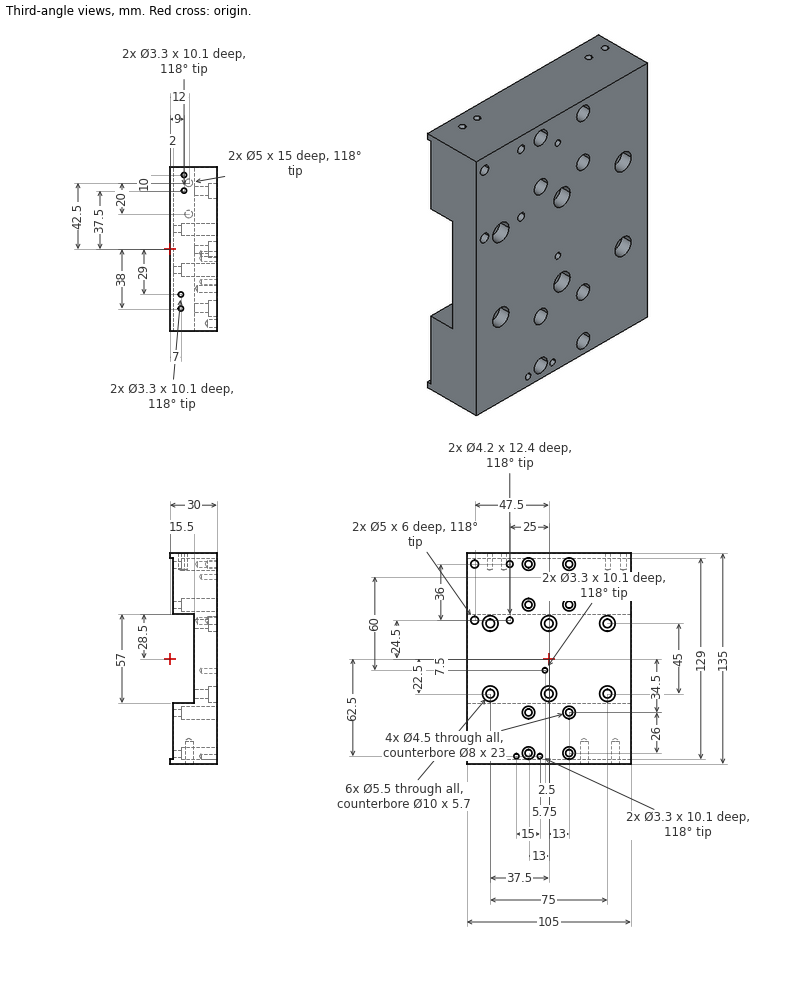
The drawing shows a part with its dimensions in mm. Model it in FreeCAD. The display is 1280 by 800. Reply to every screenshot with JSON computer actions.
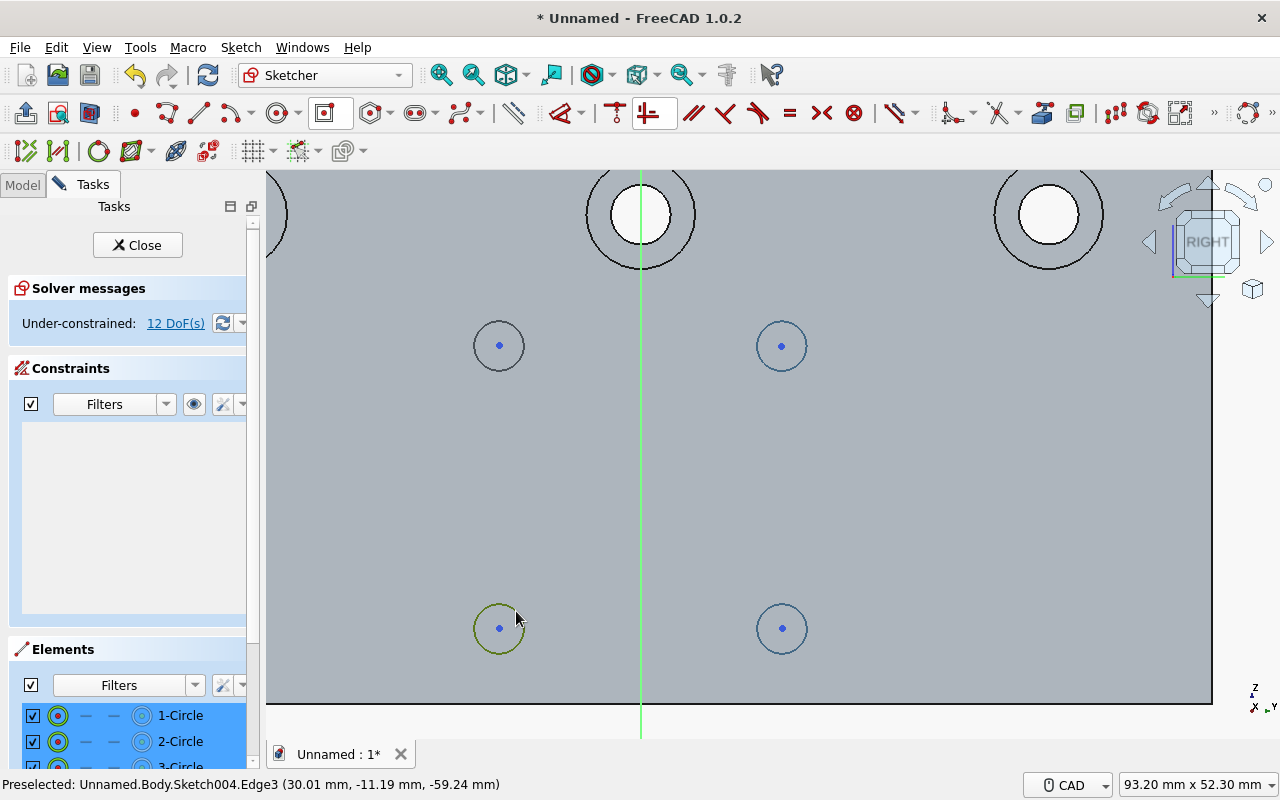
{"action": "left_click", "coordinate": [516, 328]}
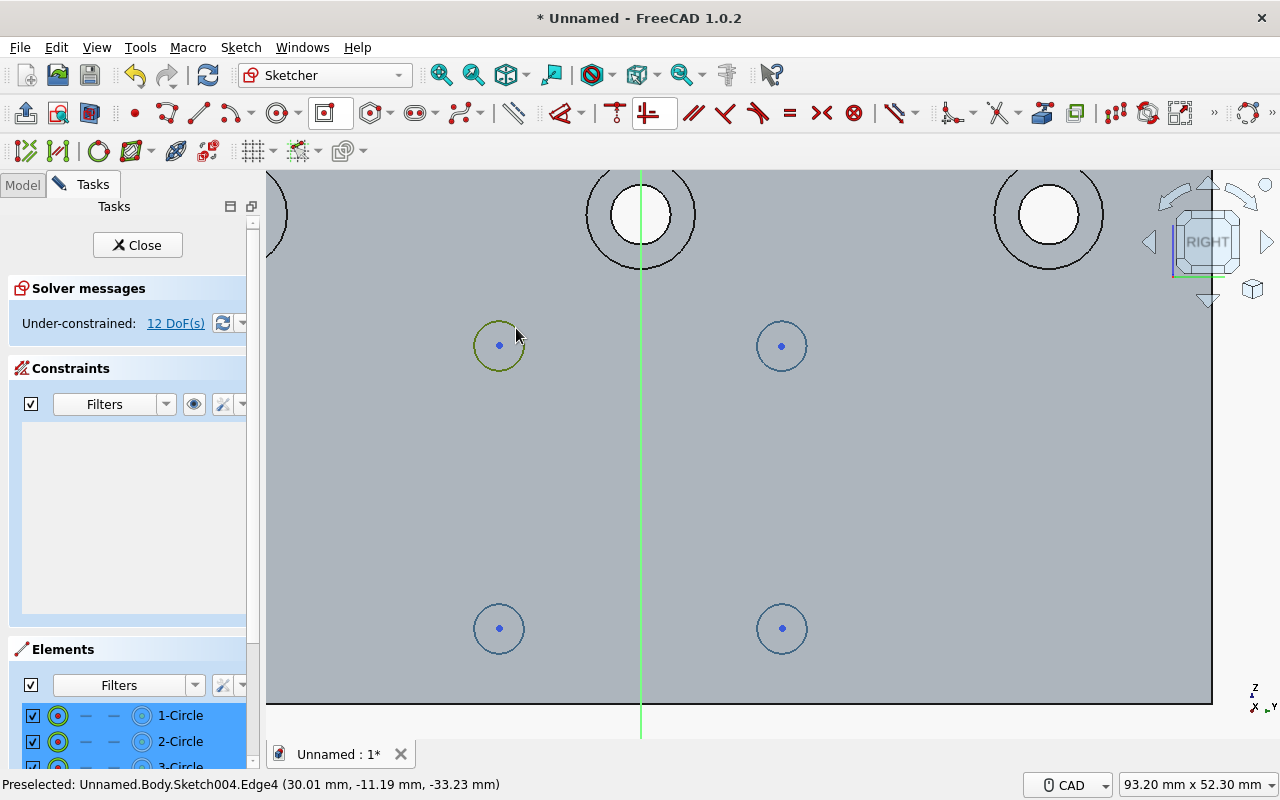
{"action": "left_click", "coordinate": [790, 114]}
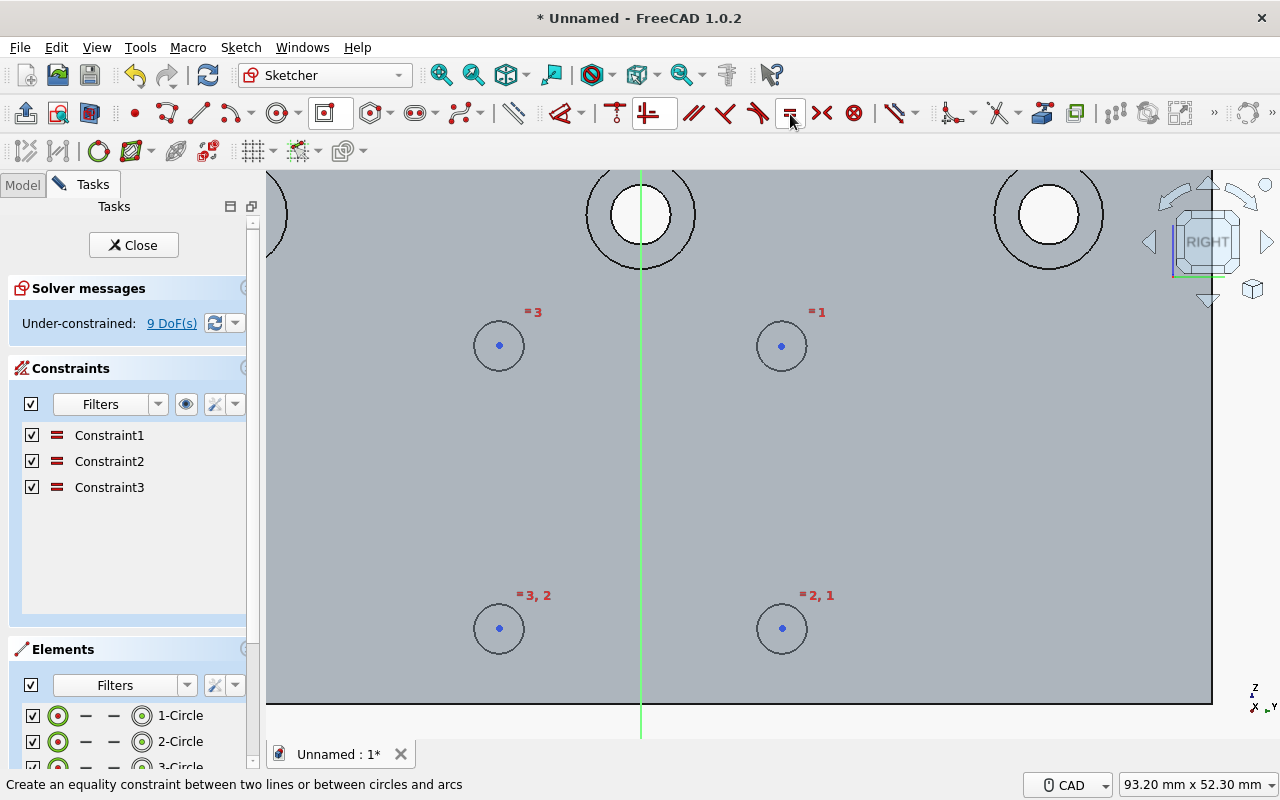
{"action": "left_click", "coordinate": [782, 346]}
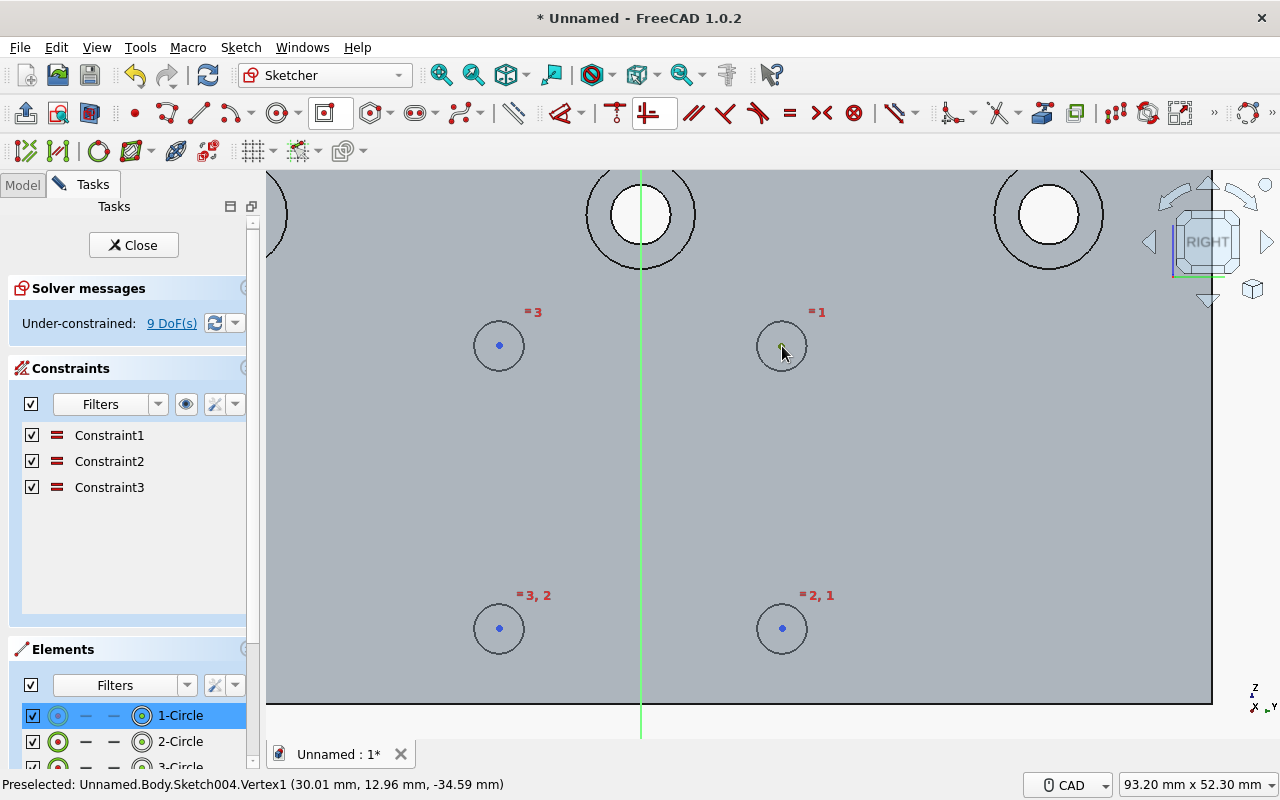
{"action": "left_click", "coordinate": [782, 629]}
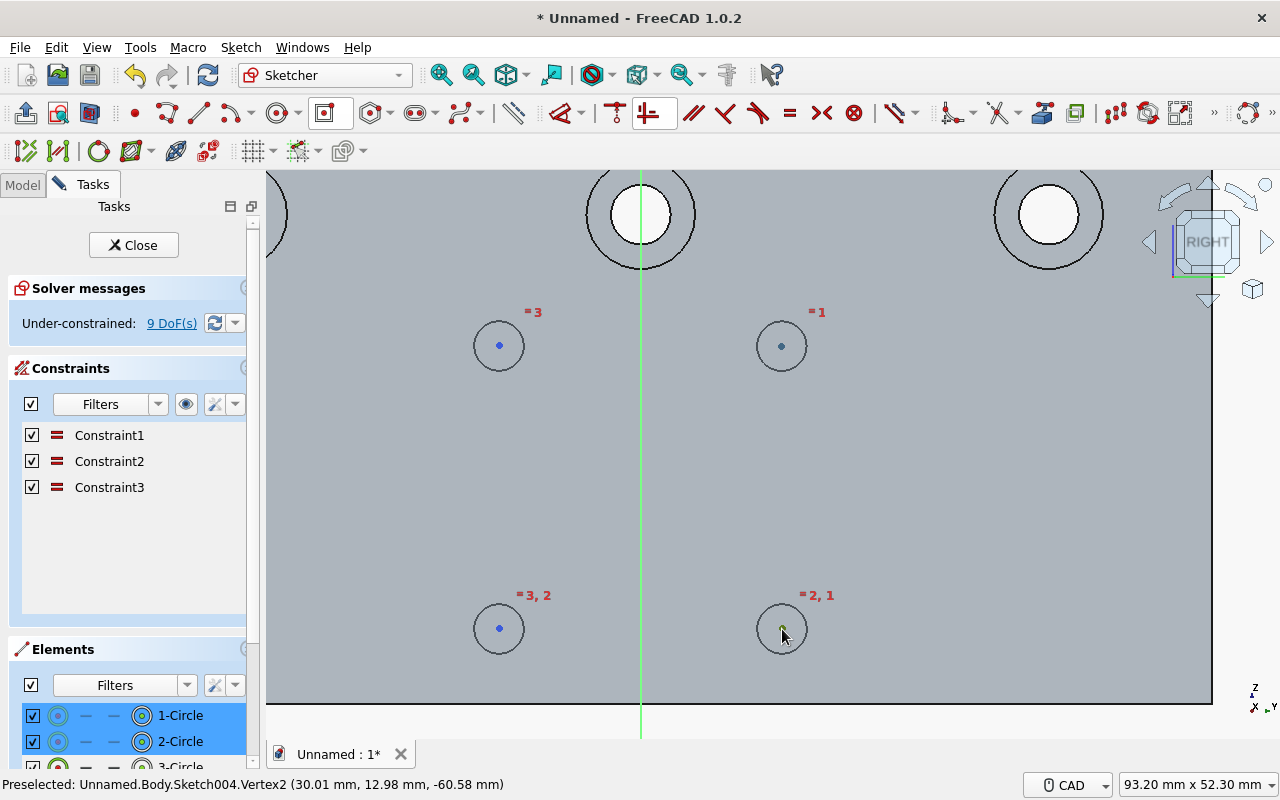
{"action": "left_click", "coordinate": [672, 114]}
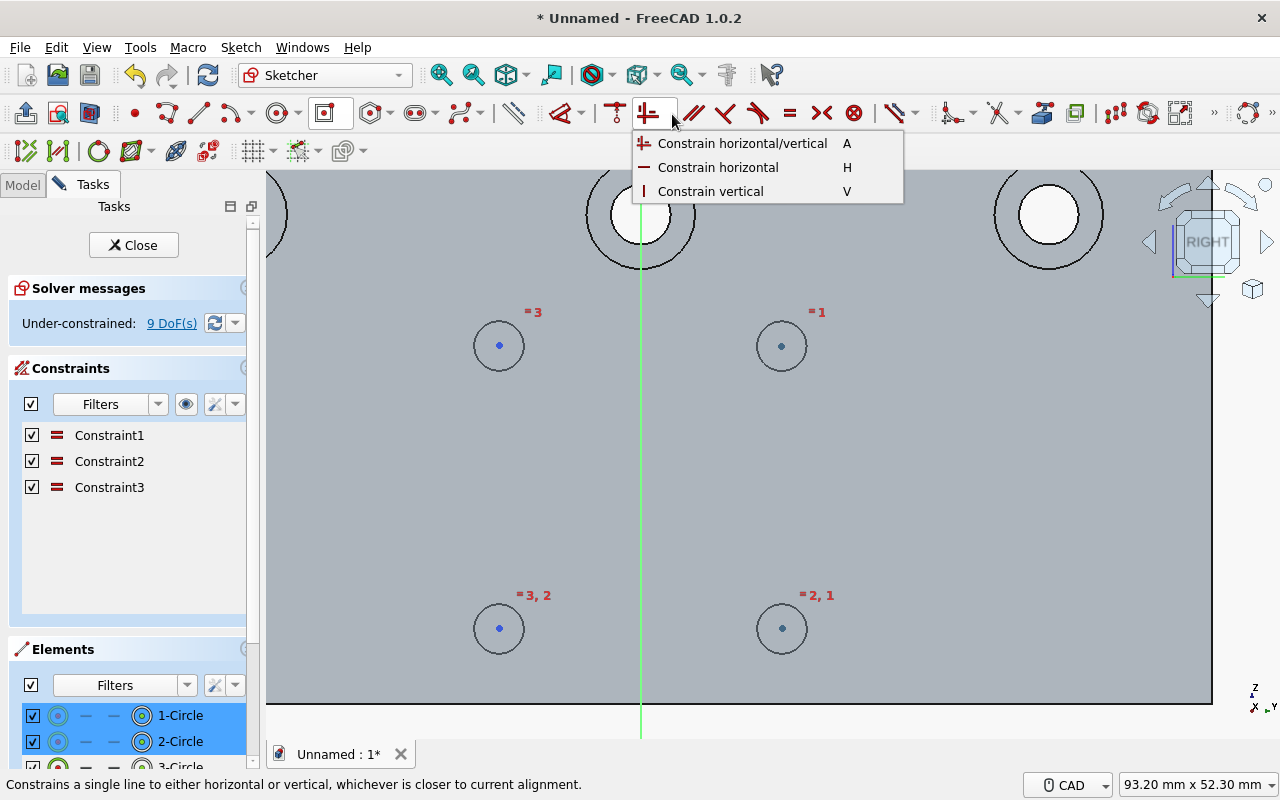
{"action": "left_click", "coordinate": [768, 191]}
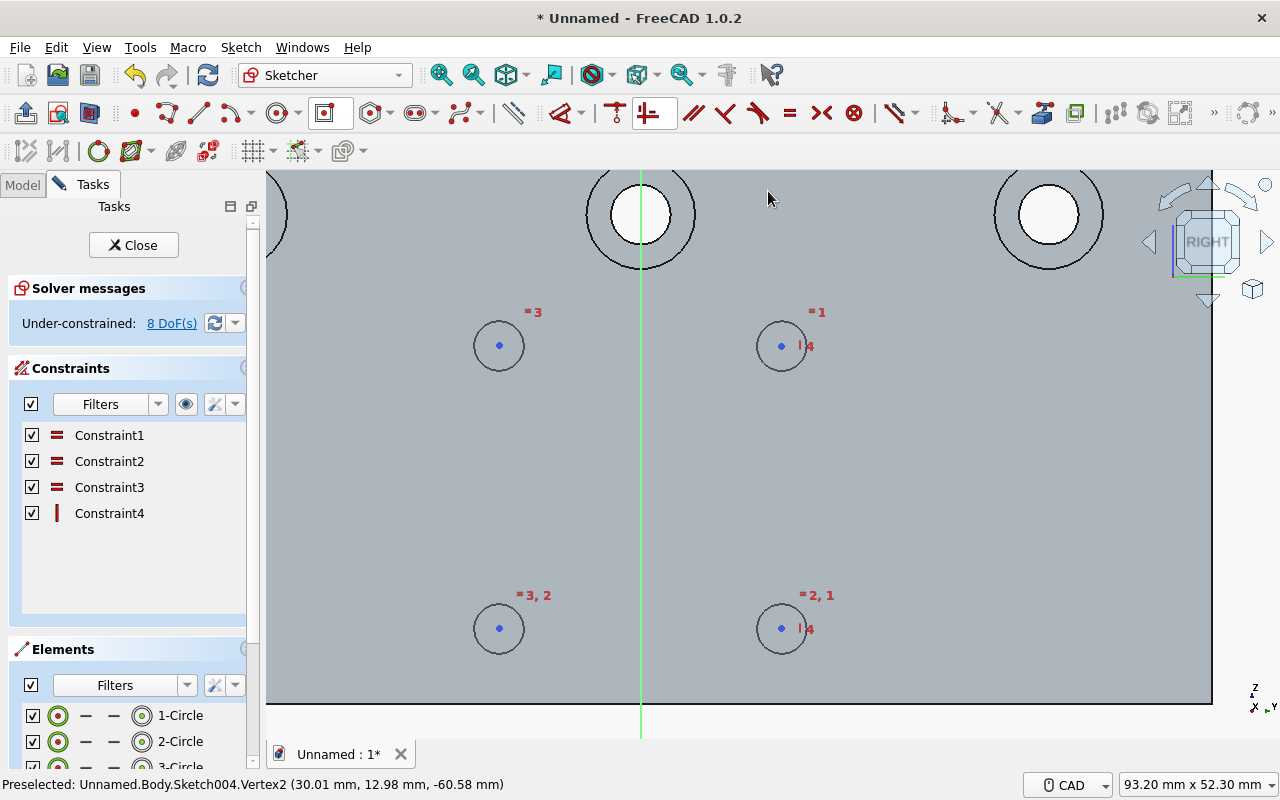
{"action": "left_click", "coordinate": [782, 629]}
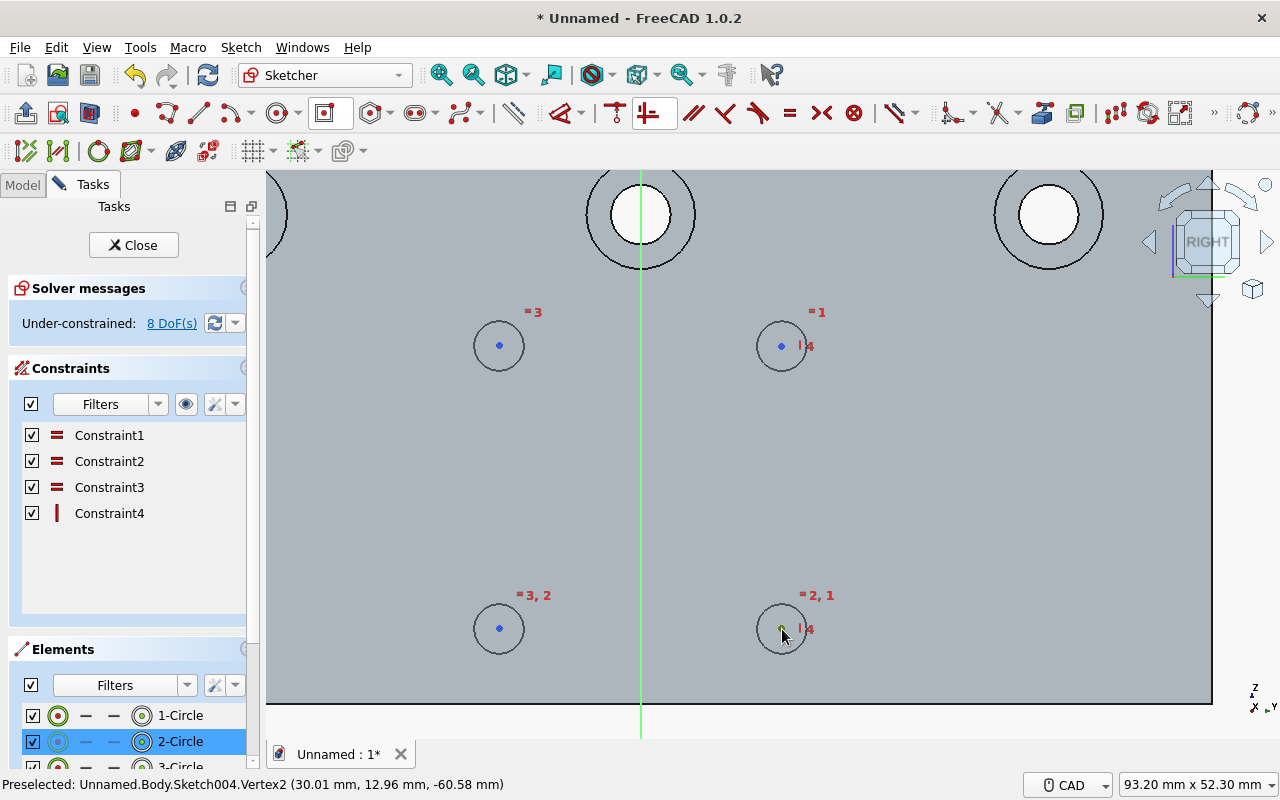
{"action": "left_click", "coordinate": [499, 629]}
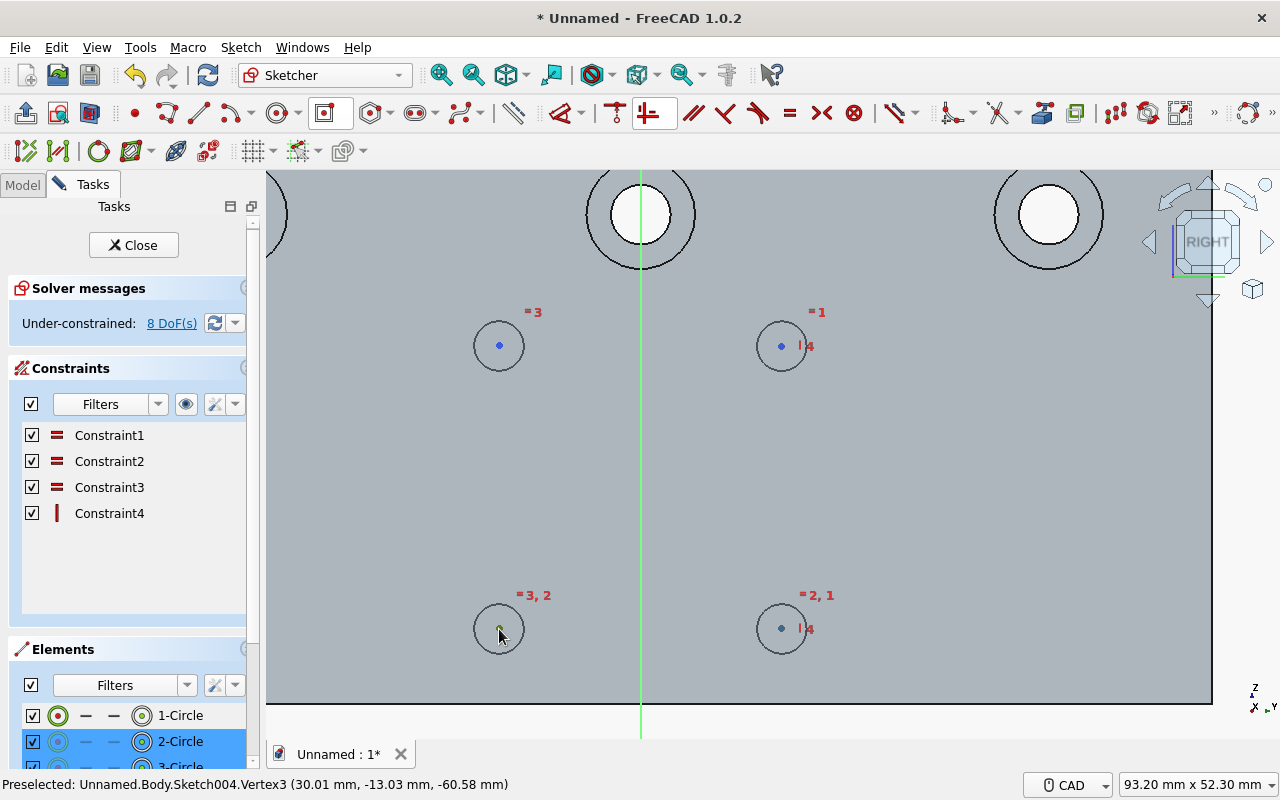
{"action": "key", "text": "h"}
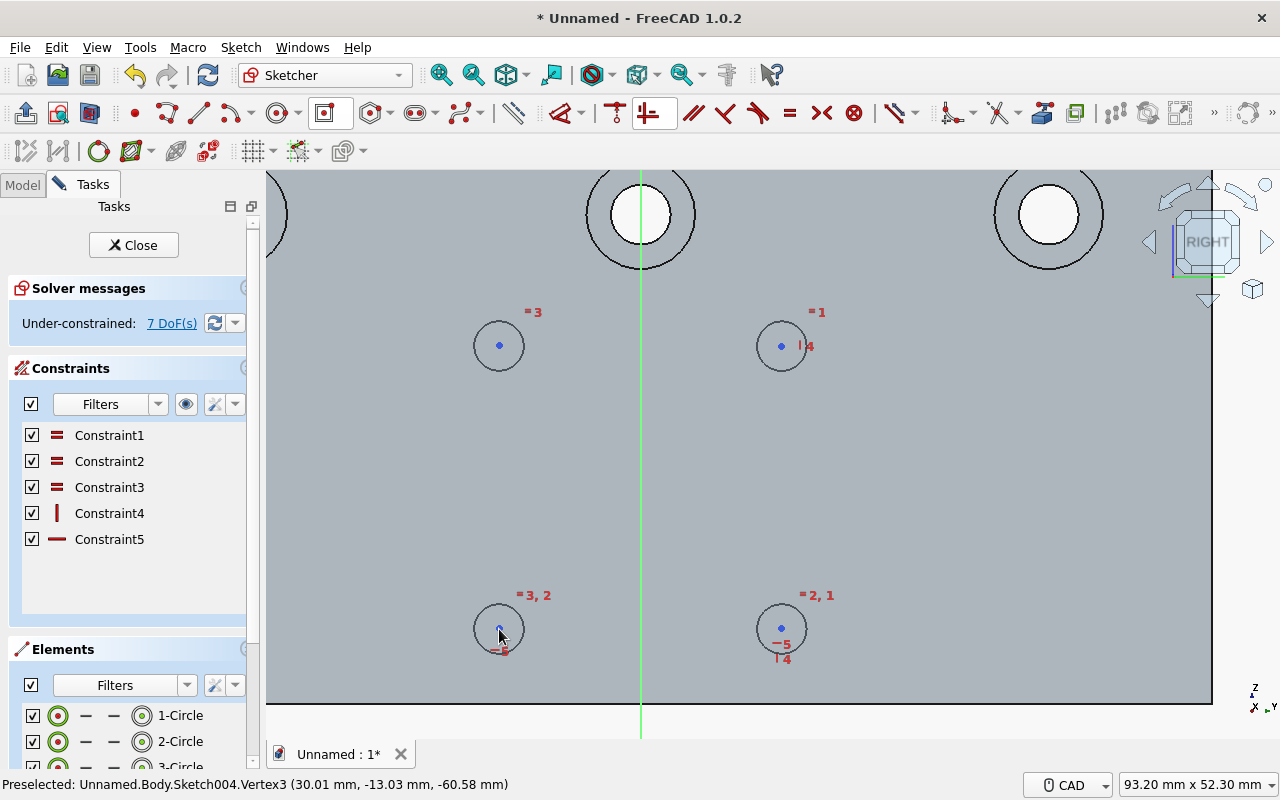
{"action": "left_click", "coordinate": [499, 629]}